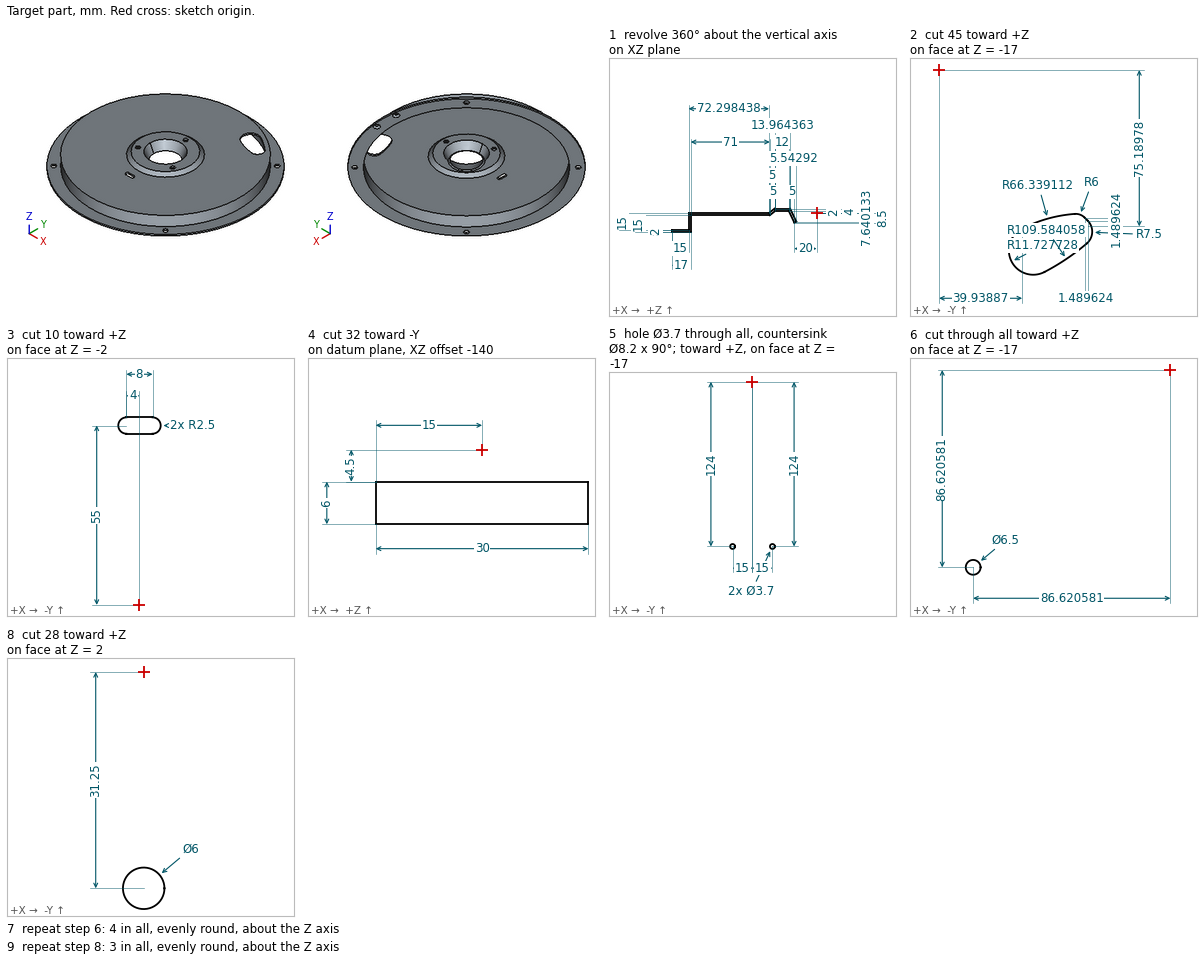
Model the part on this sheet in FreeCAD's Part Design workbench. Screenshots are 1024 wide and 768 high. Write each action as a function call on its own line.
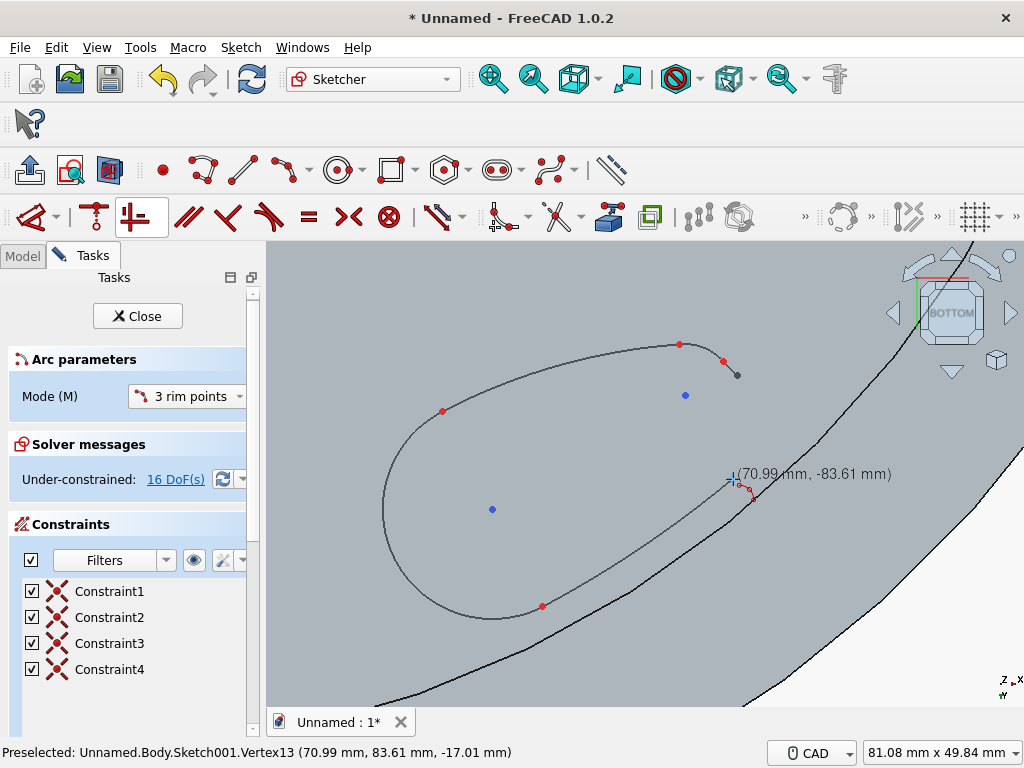
scroll(737, 374, up, 3)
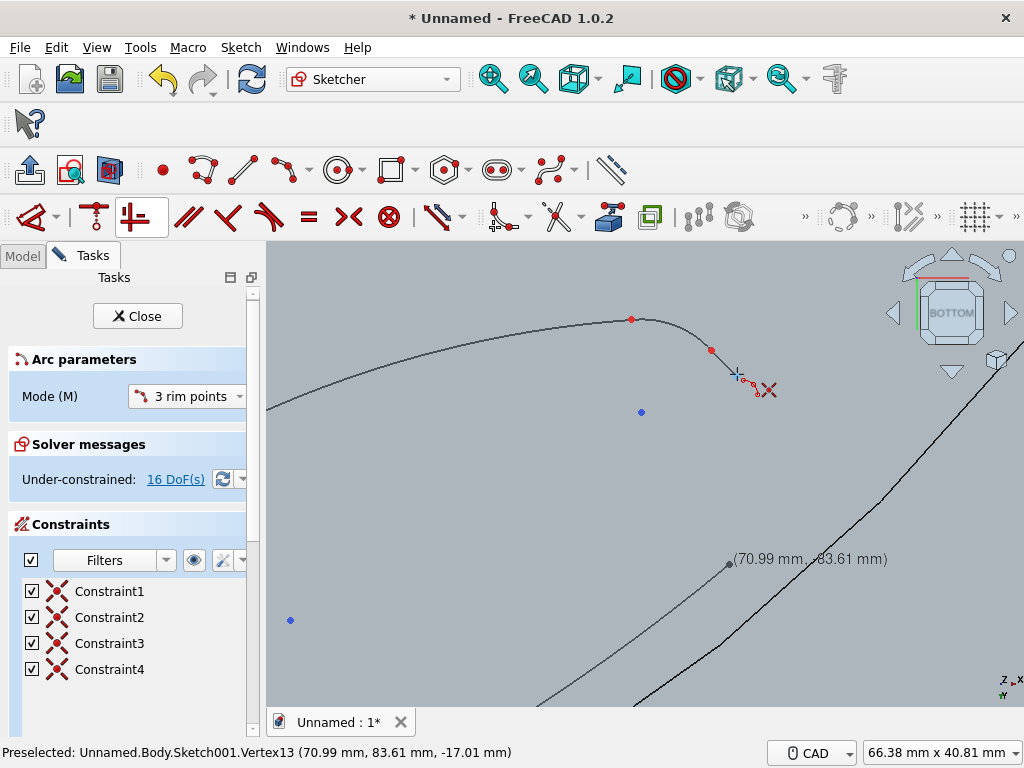
click(737, 376)
click(775, 470)
key(Escape)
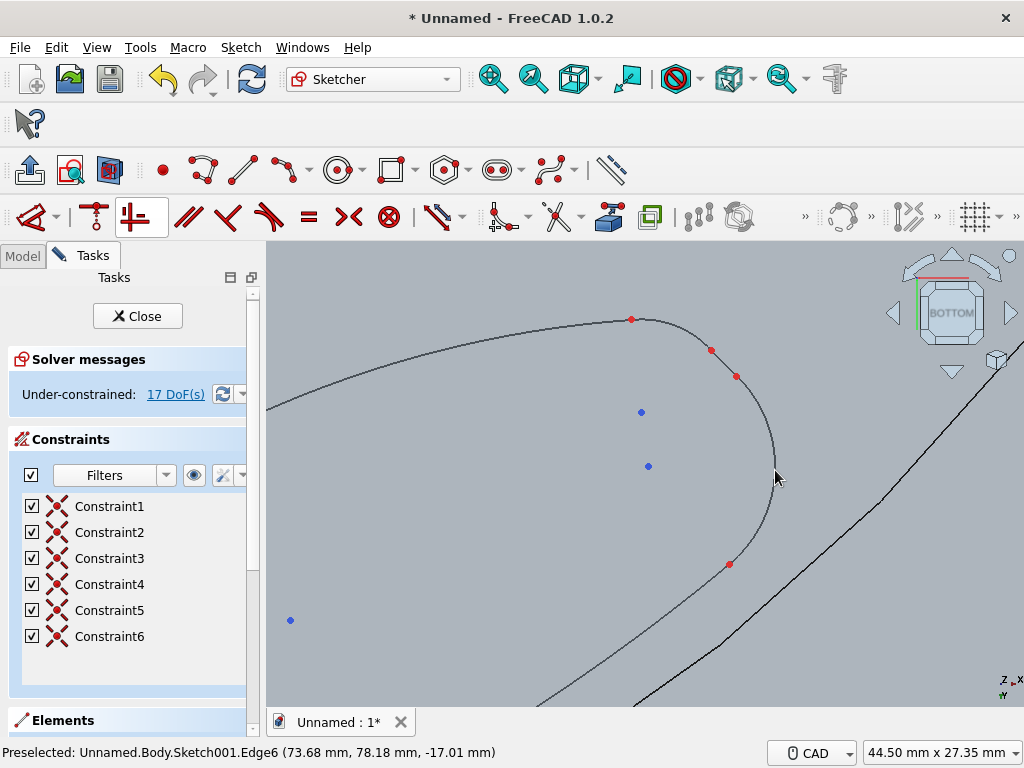
scroll(729, 368, up, 2)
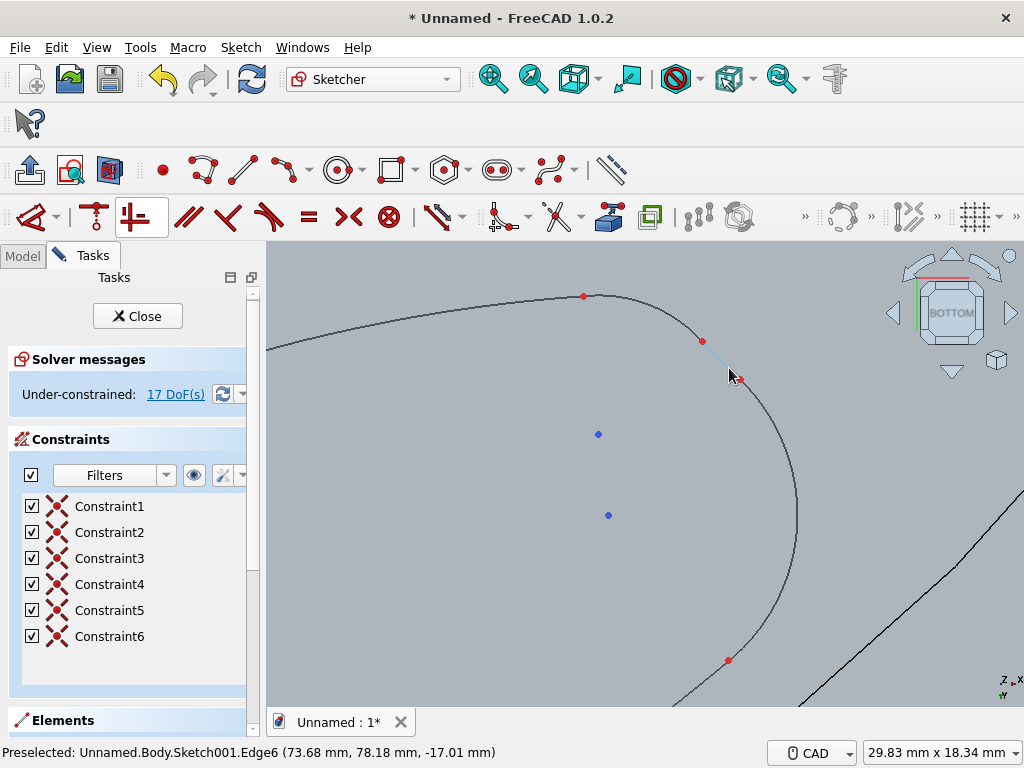
click(729, 369)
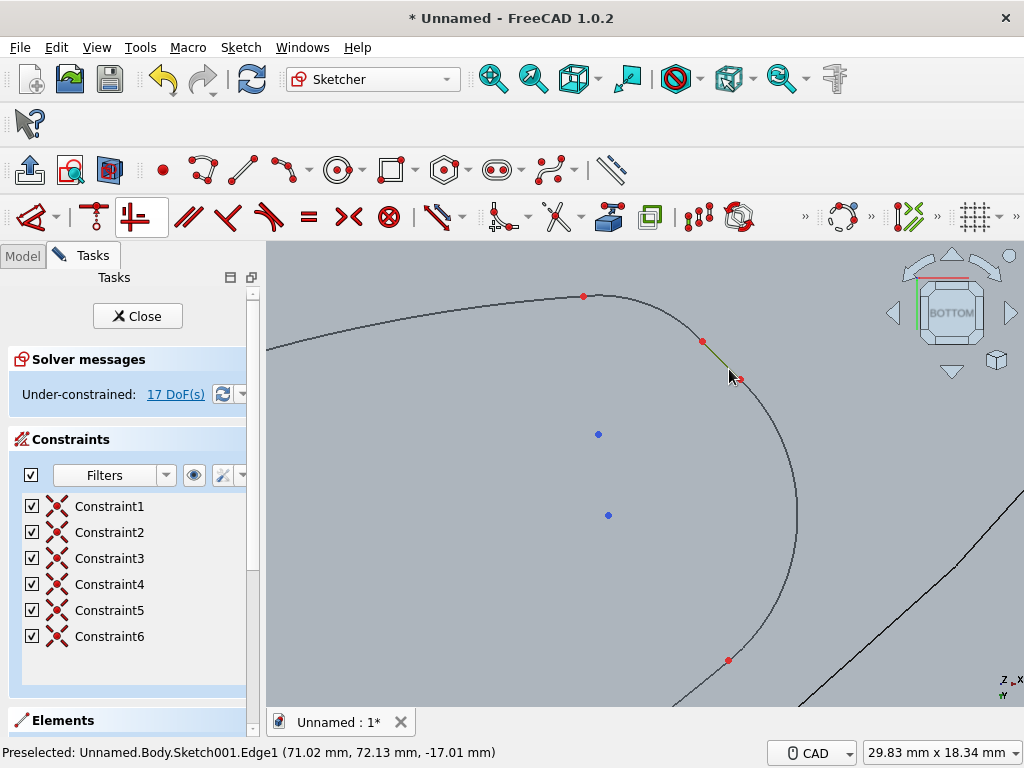
click(672, 317)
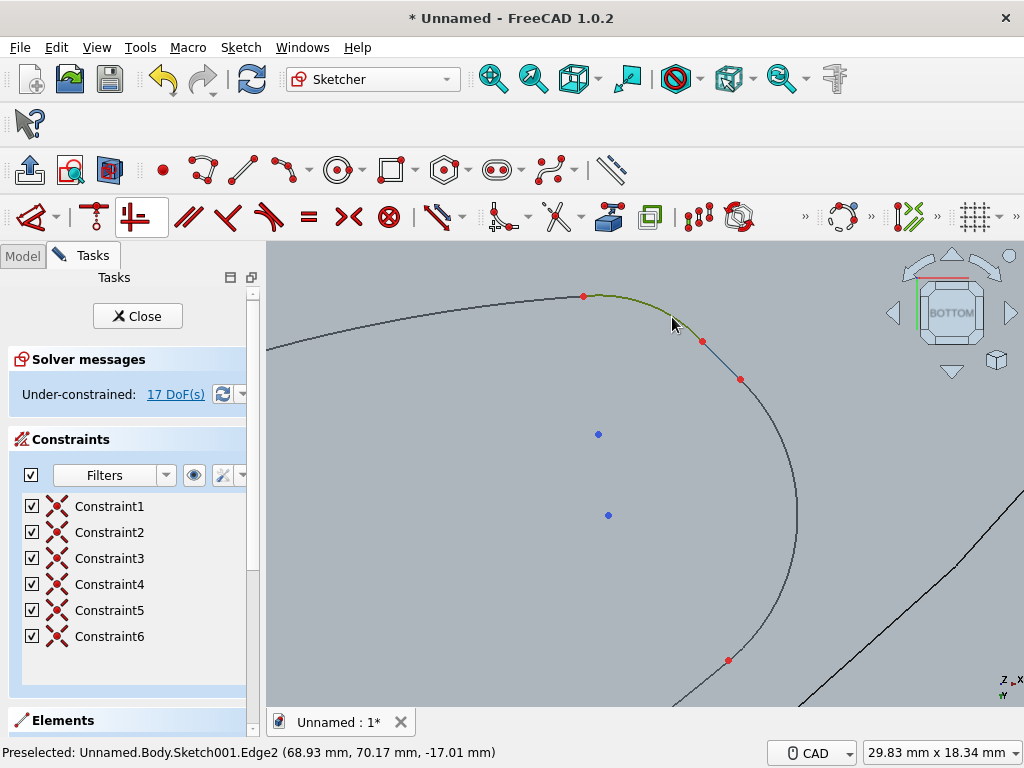
click(270, 218)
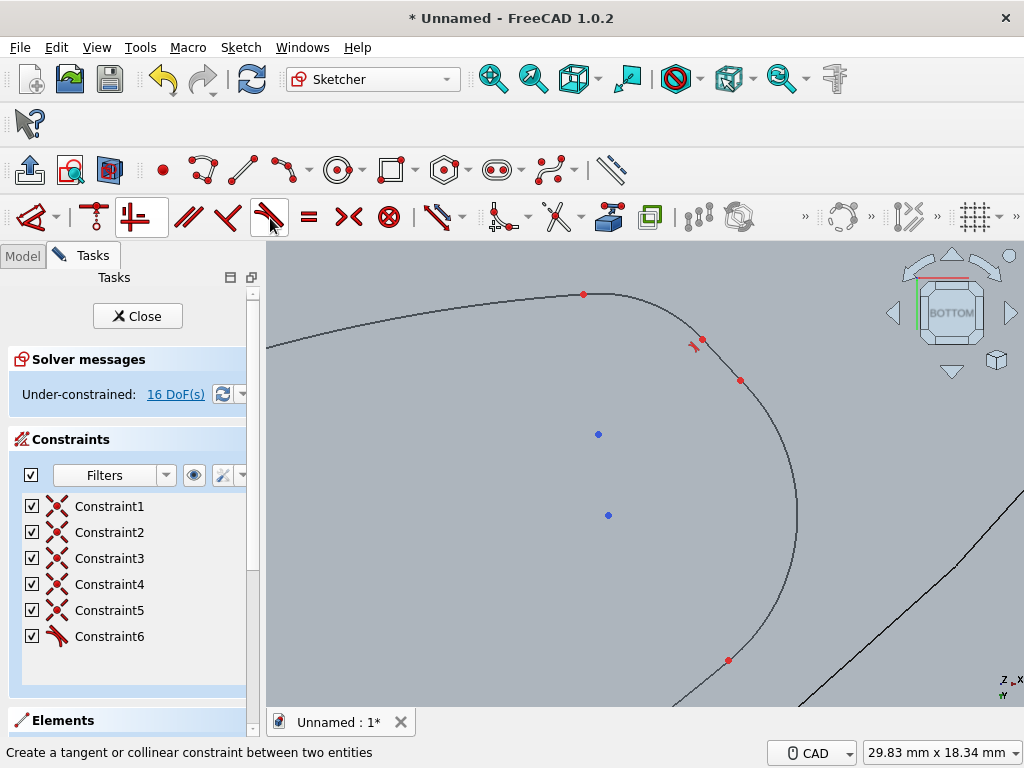
click(729, 368)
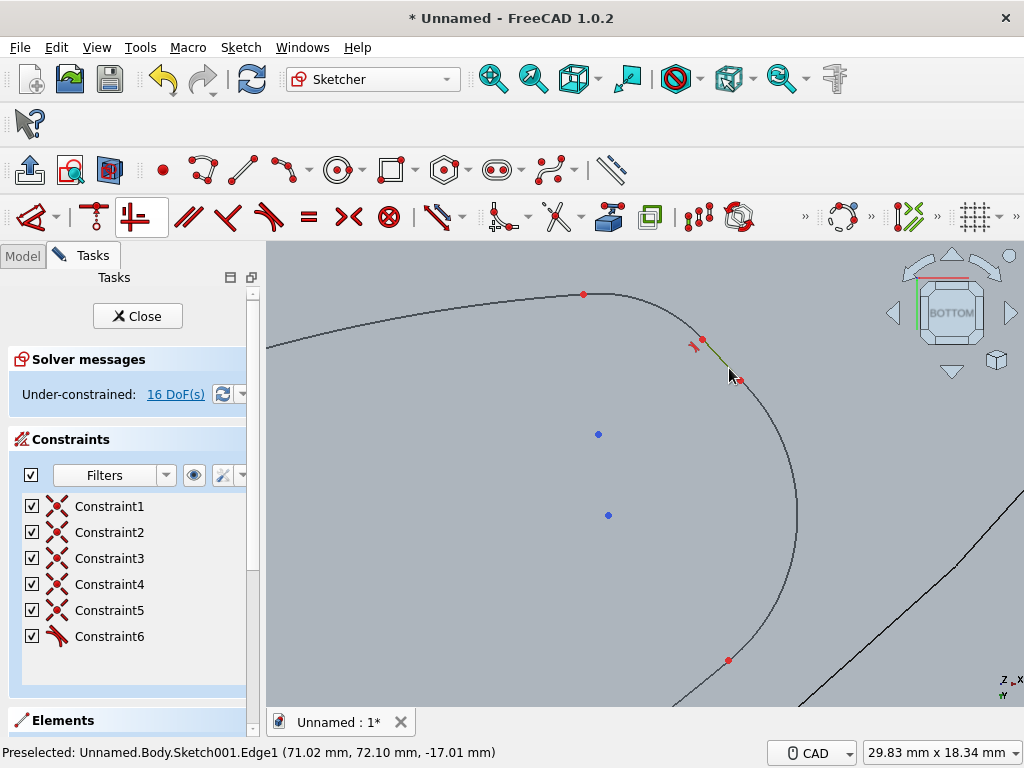
click(784, 585)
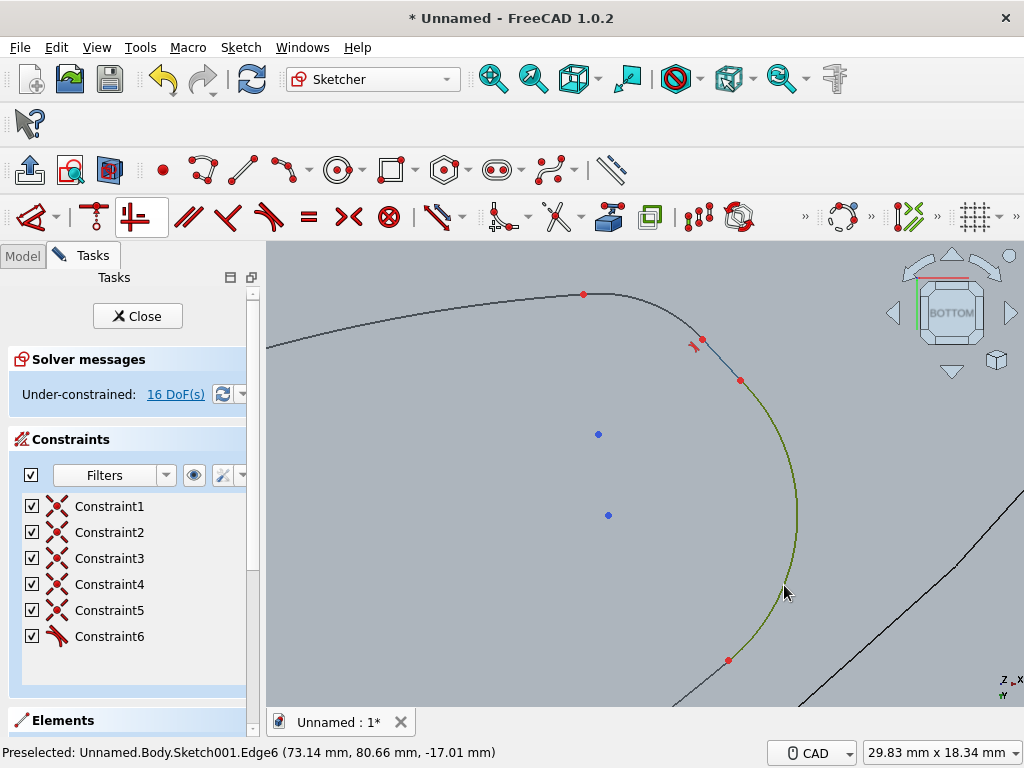
key(t)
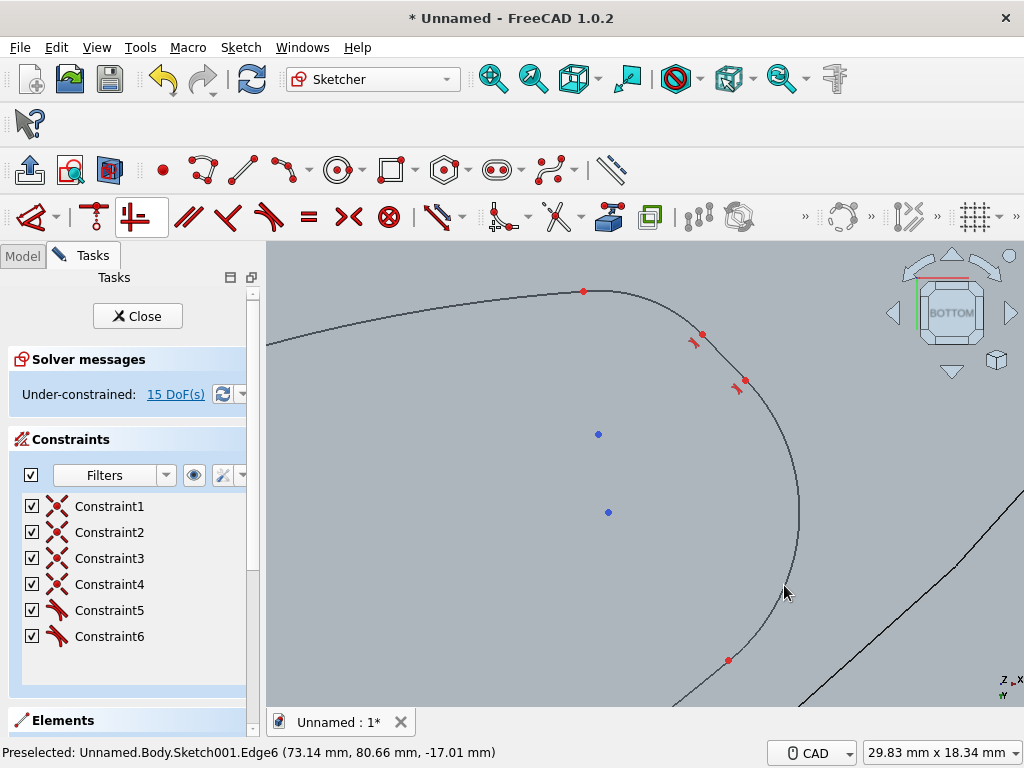
click(672, 311)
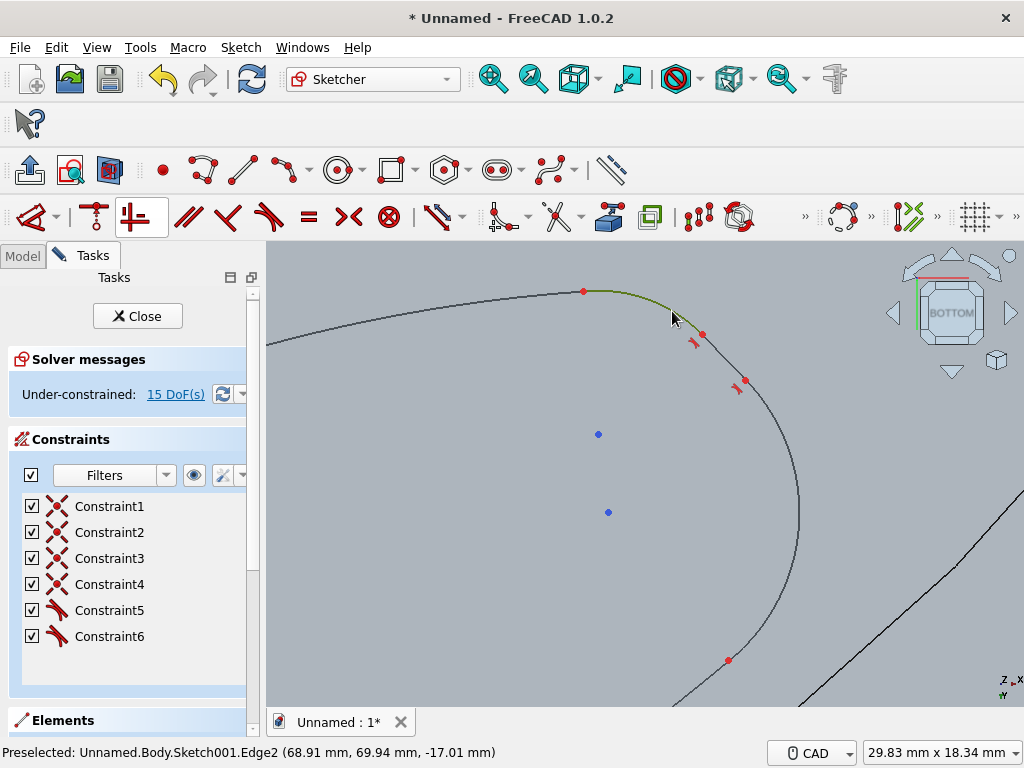
click(384, 318)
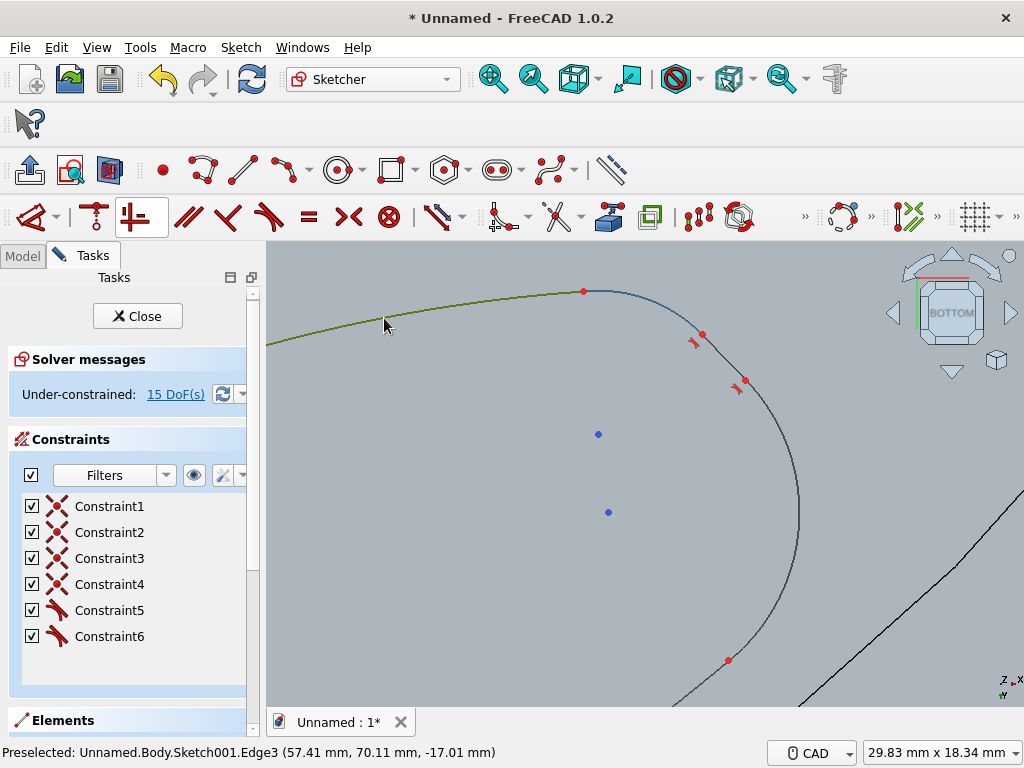
click(270, 218)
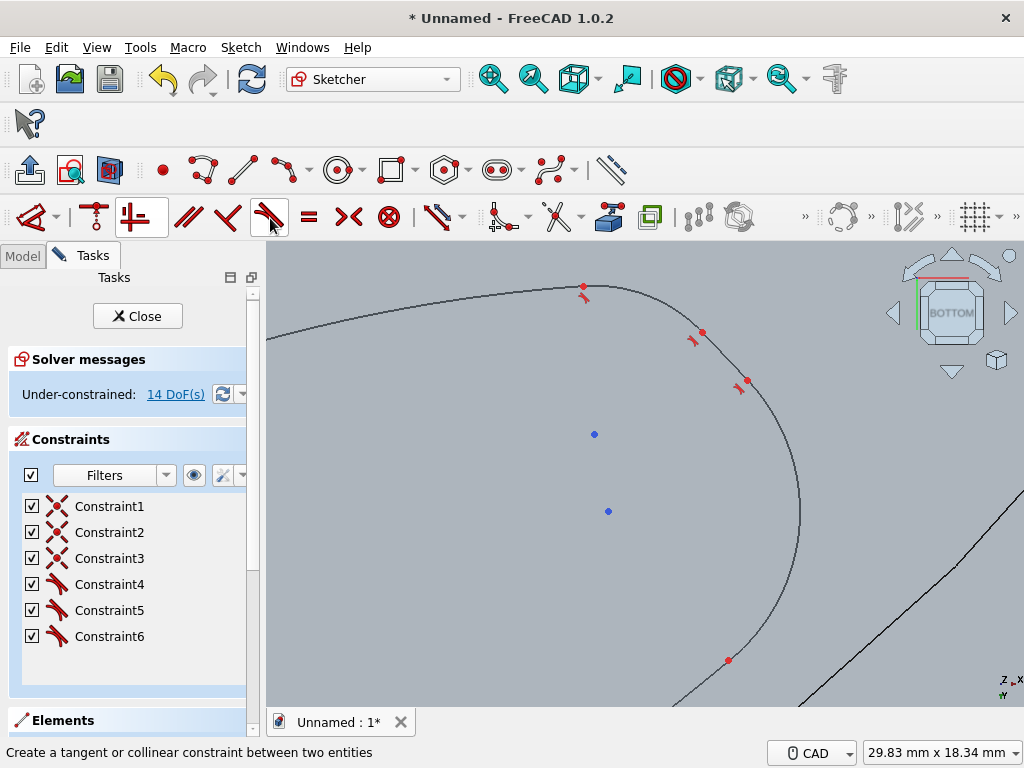
click(384, 312)